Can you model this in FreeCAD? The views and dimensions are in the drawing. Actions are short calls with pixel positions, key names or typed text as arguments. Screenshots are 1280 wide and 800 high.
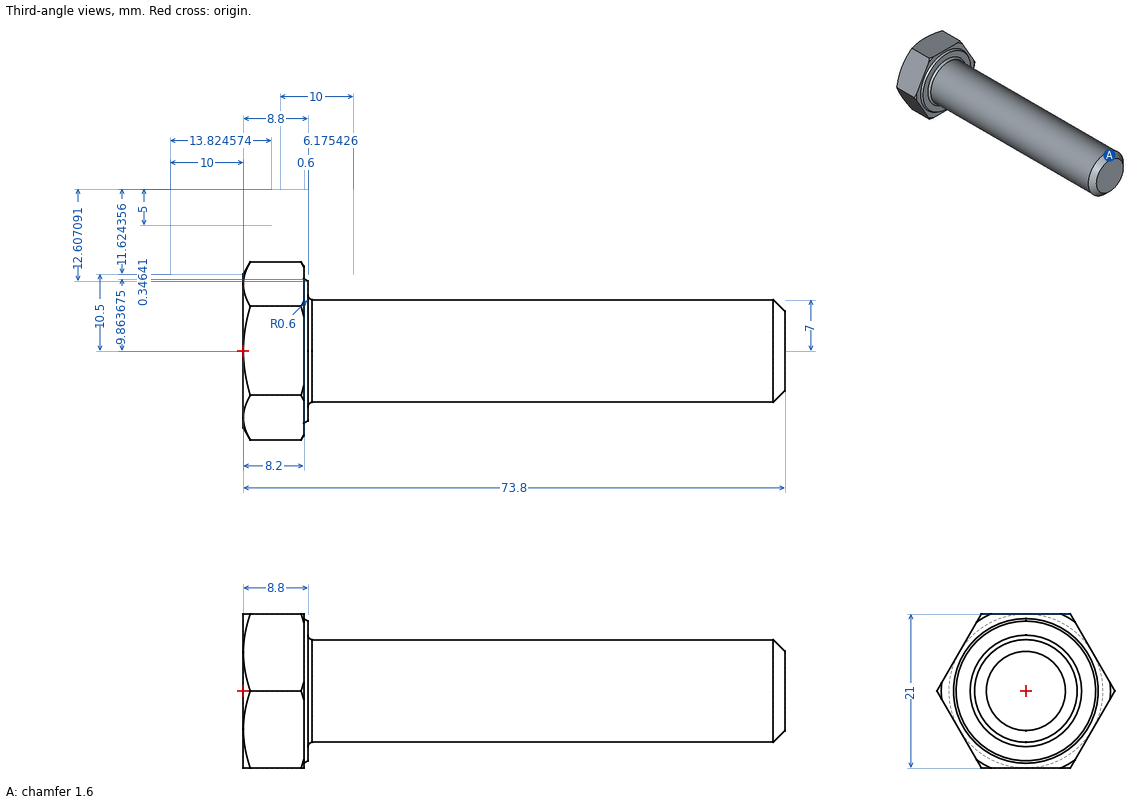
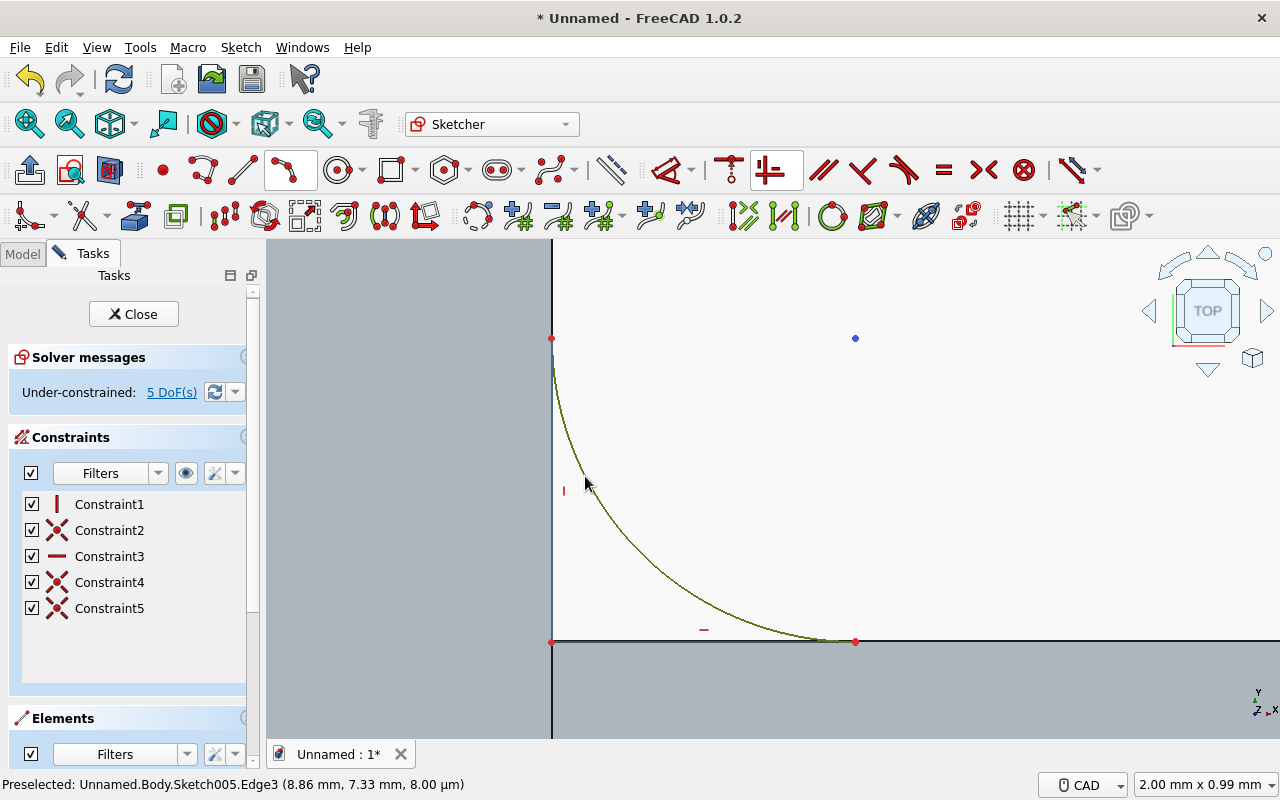
click(904, 170)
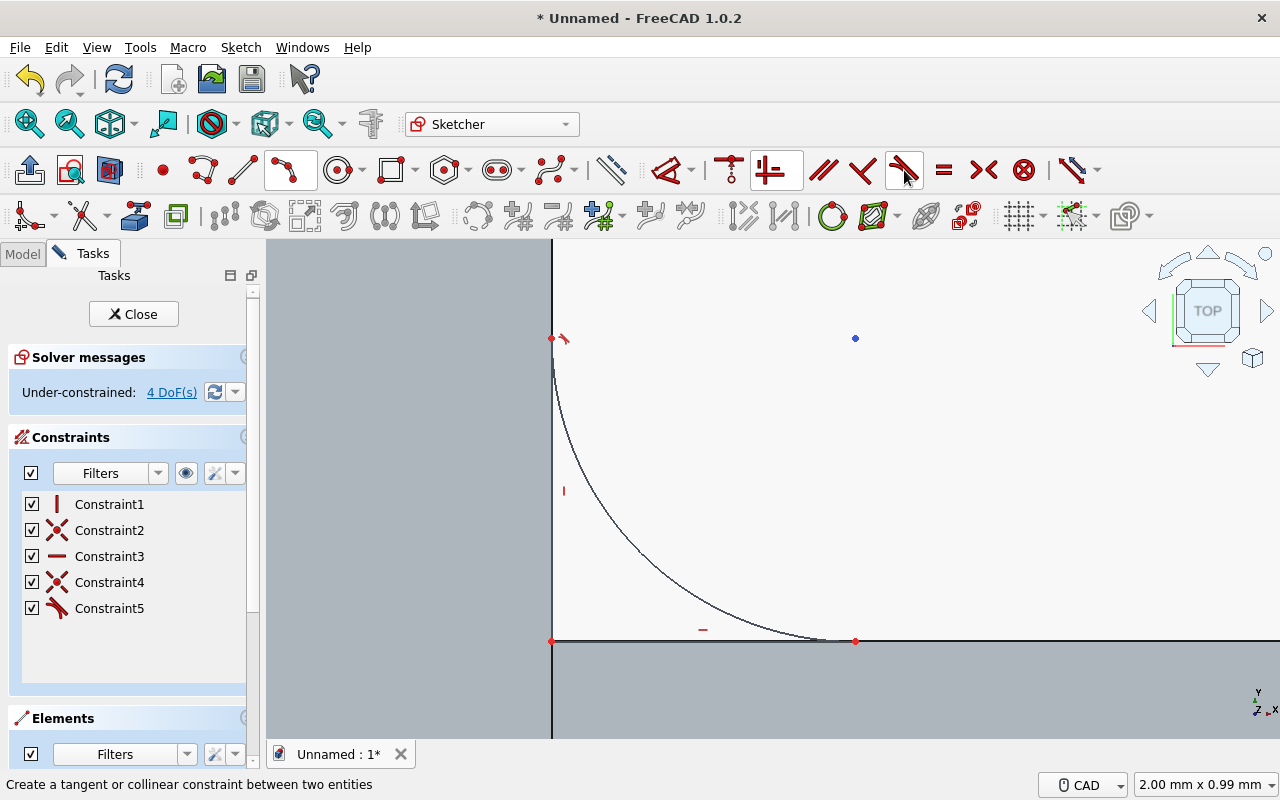
click(643, 642)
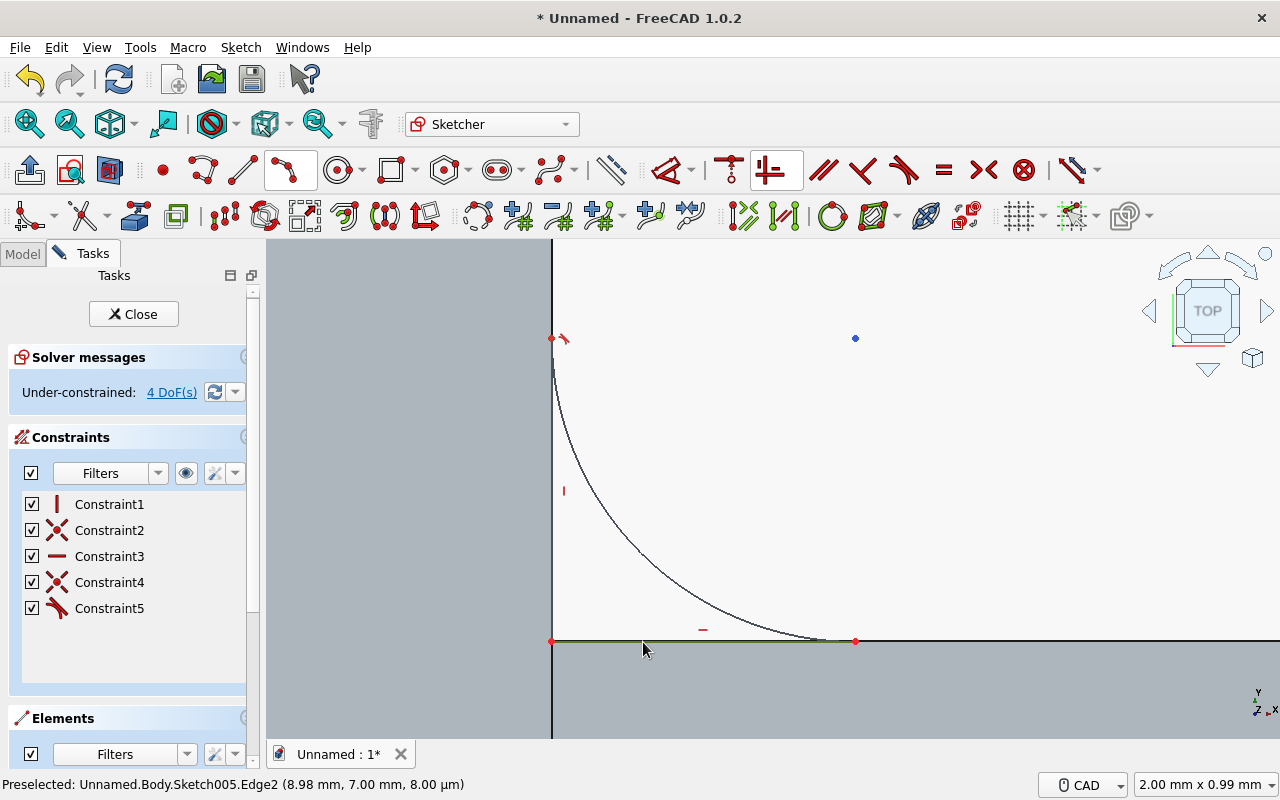
click(585, 476)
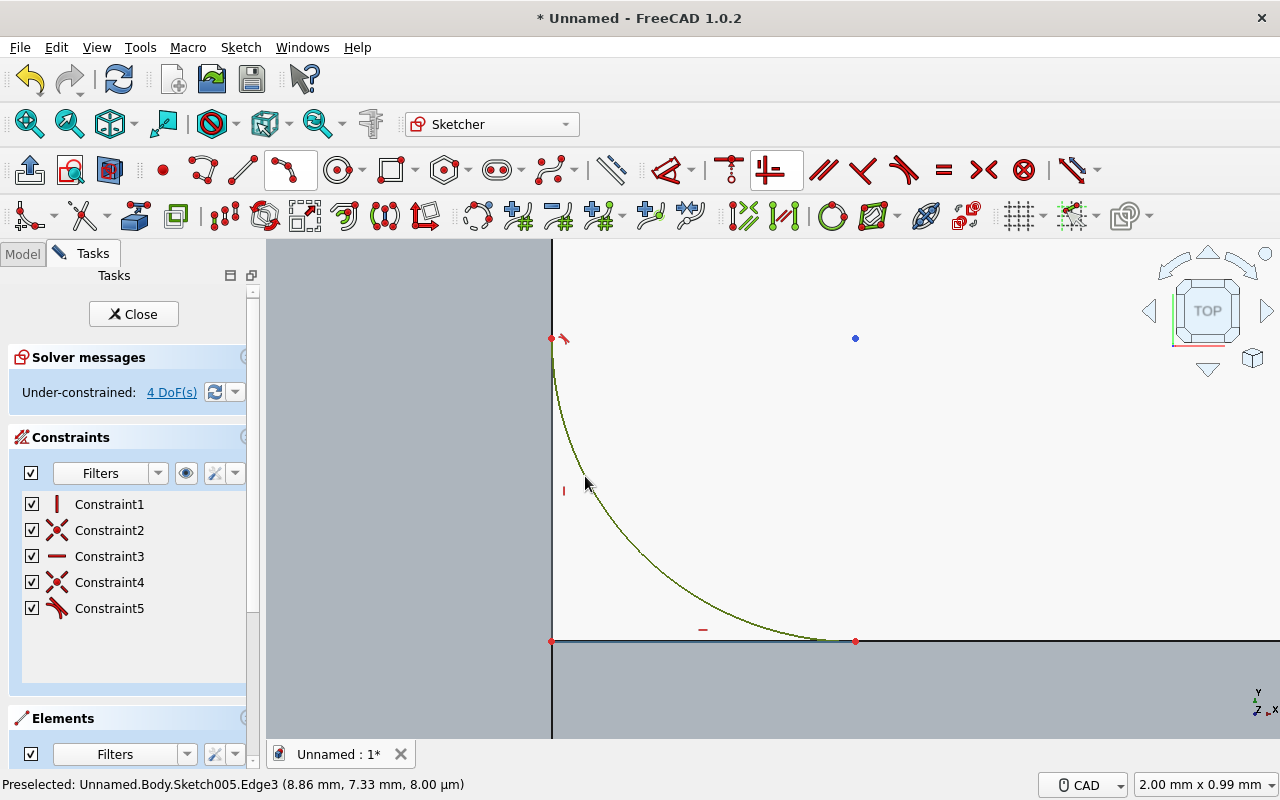
click(904, 170)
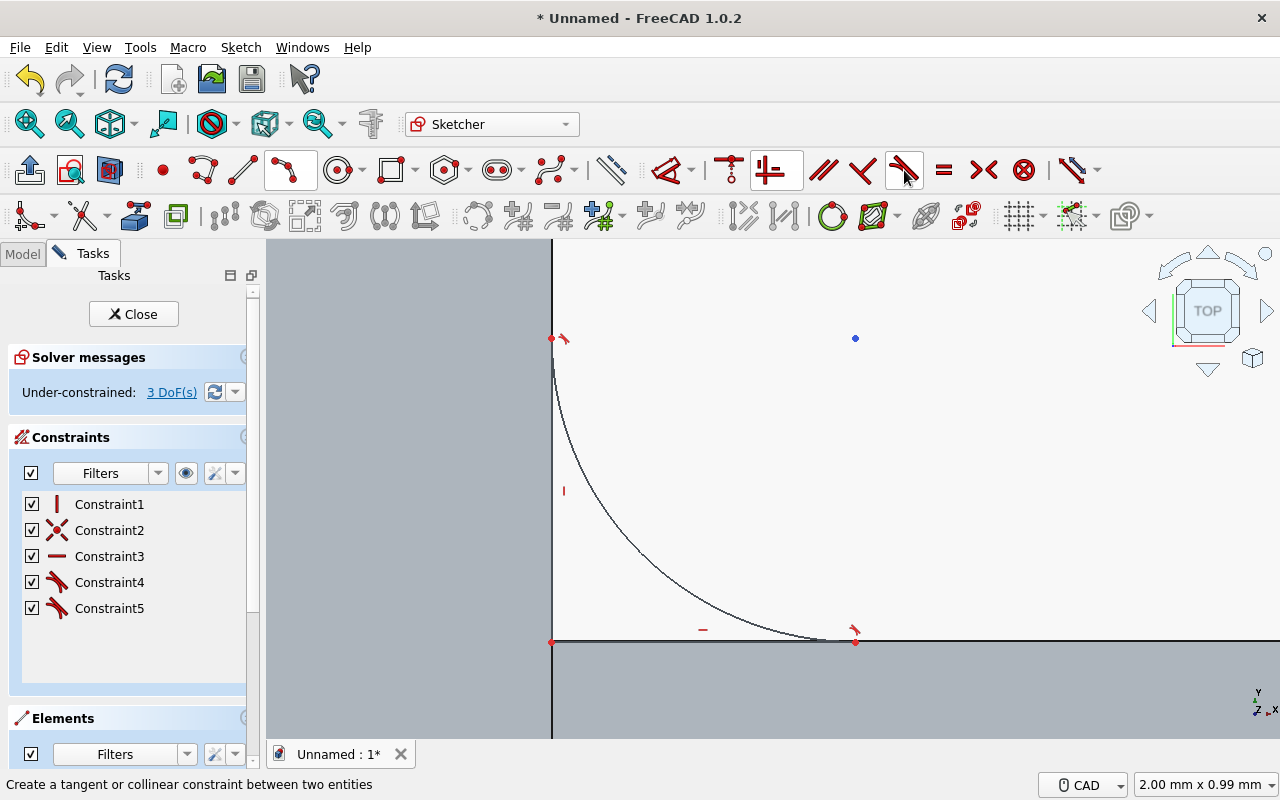
click(666, 170)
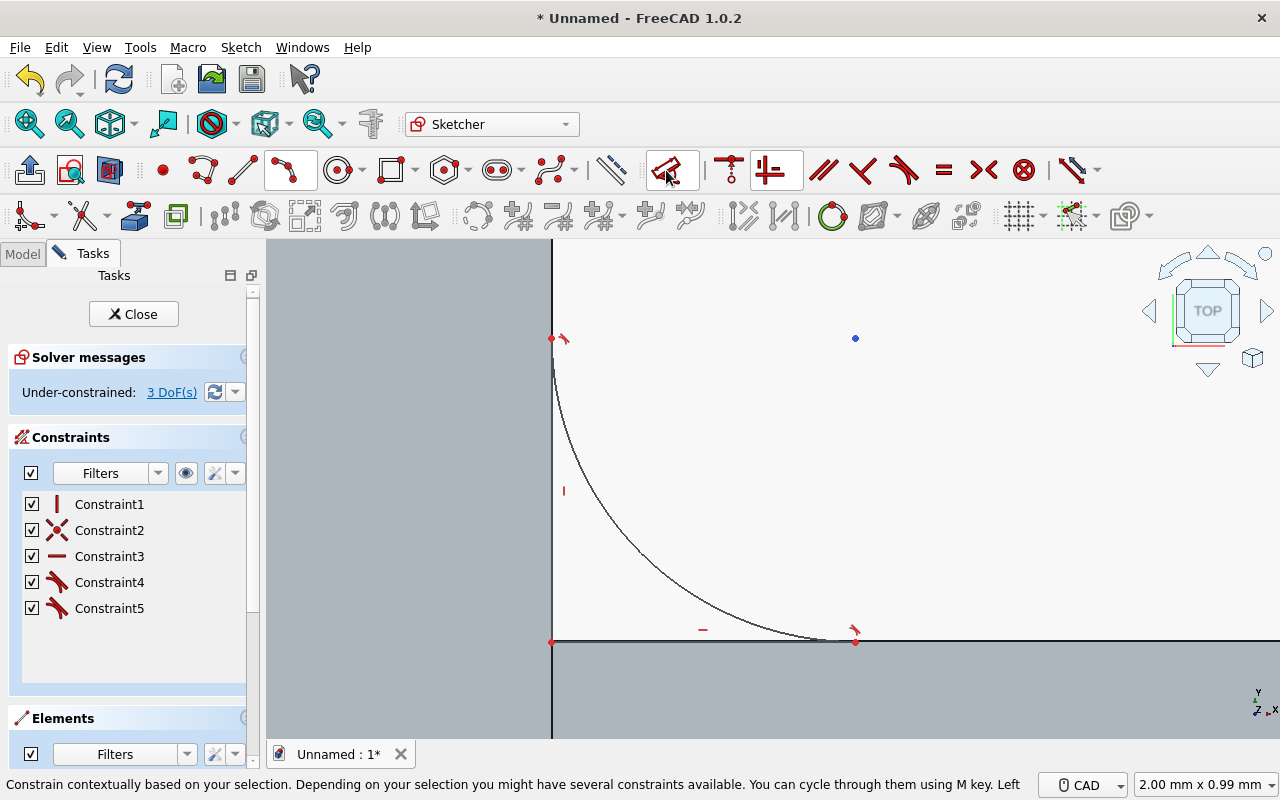
click(585, 476)
click(520, 328)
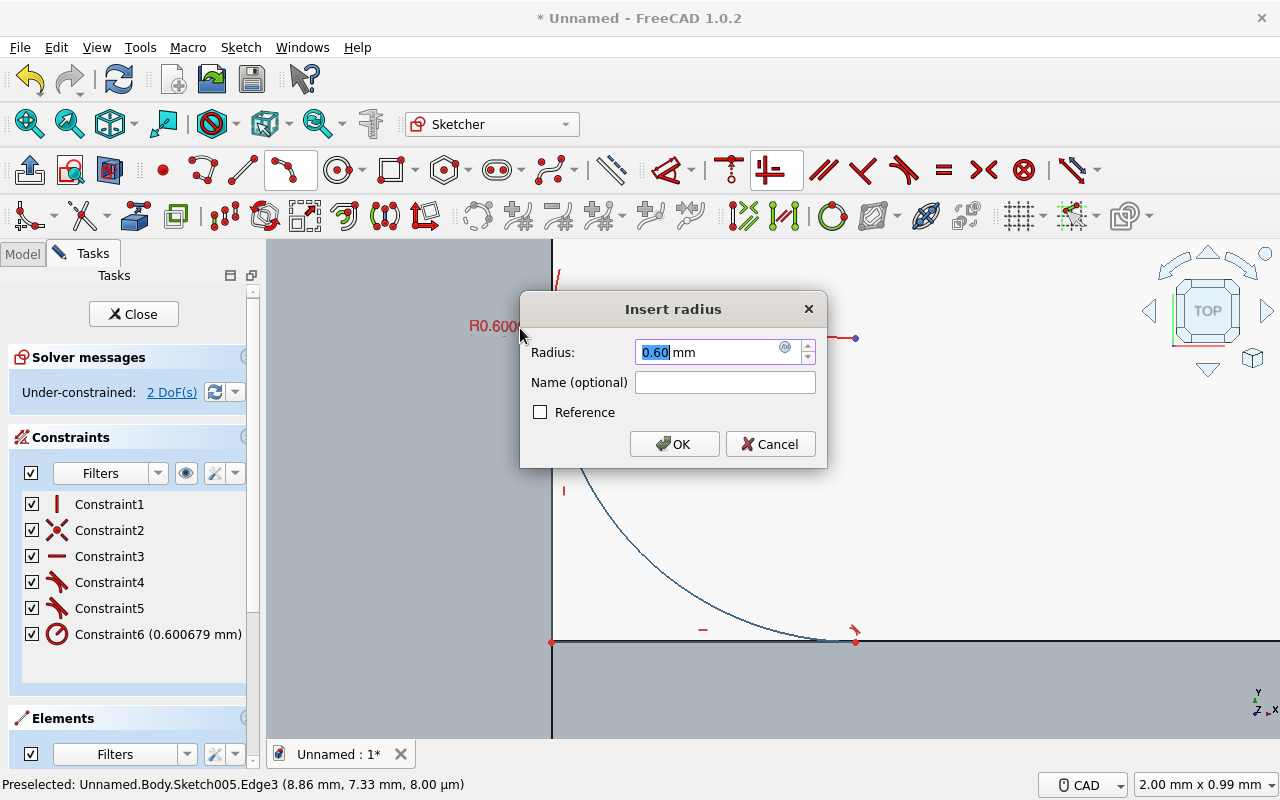
text(0.6)
key(Return)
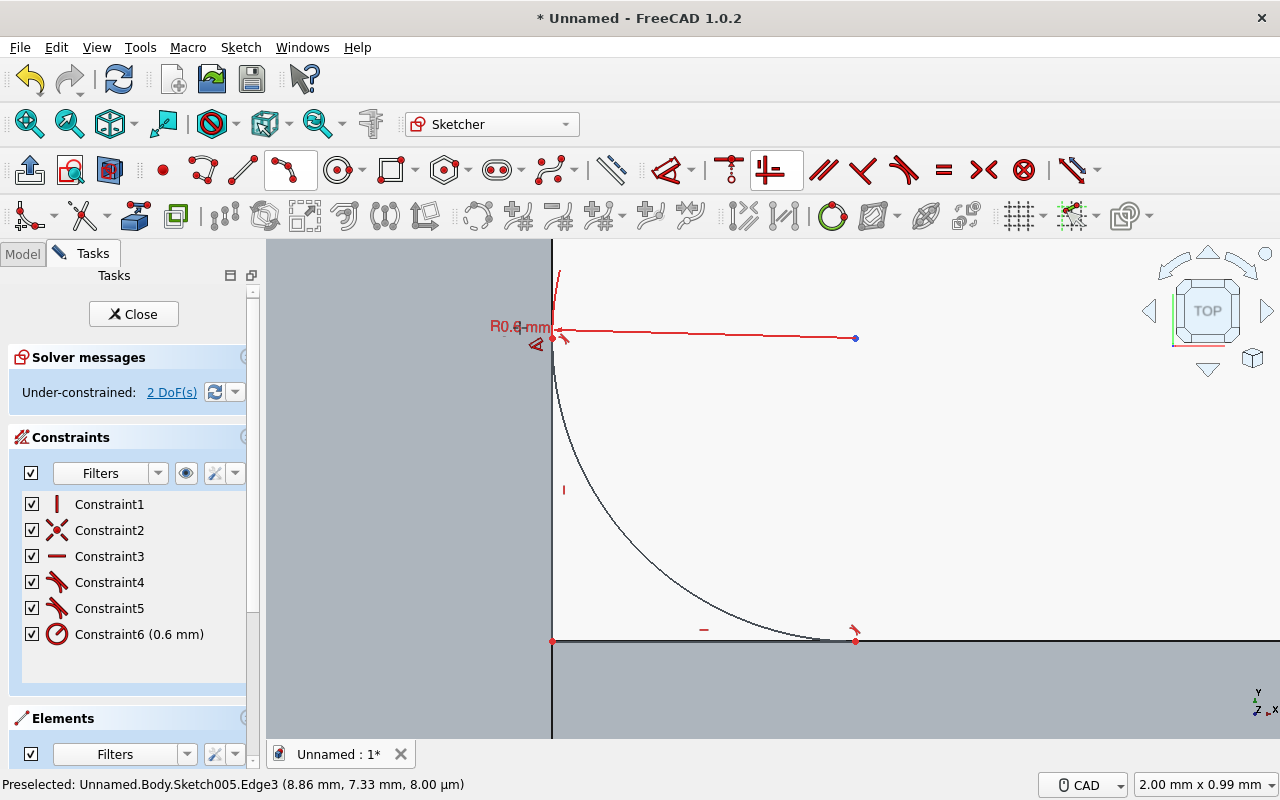
click(552, 642)
click(586, 676)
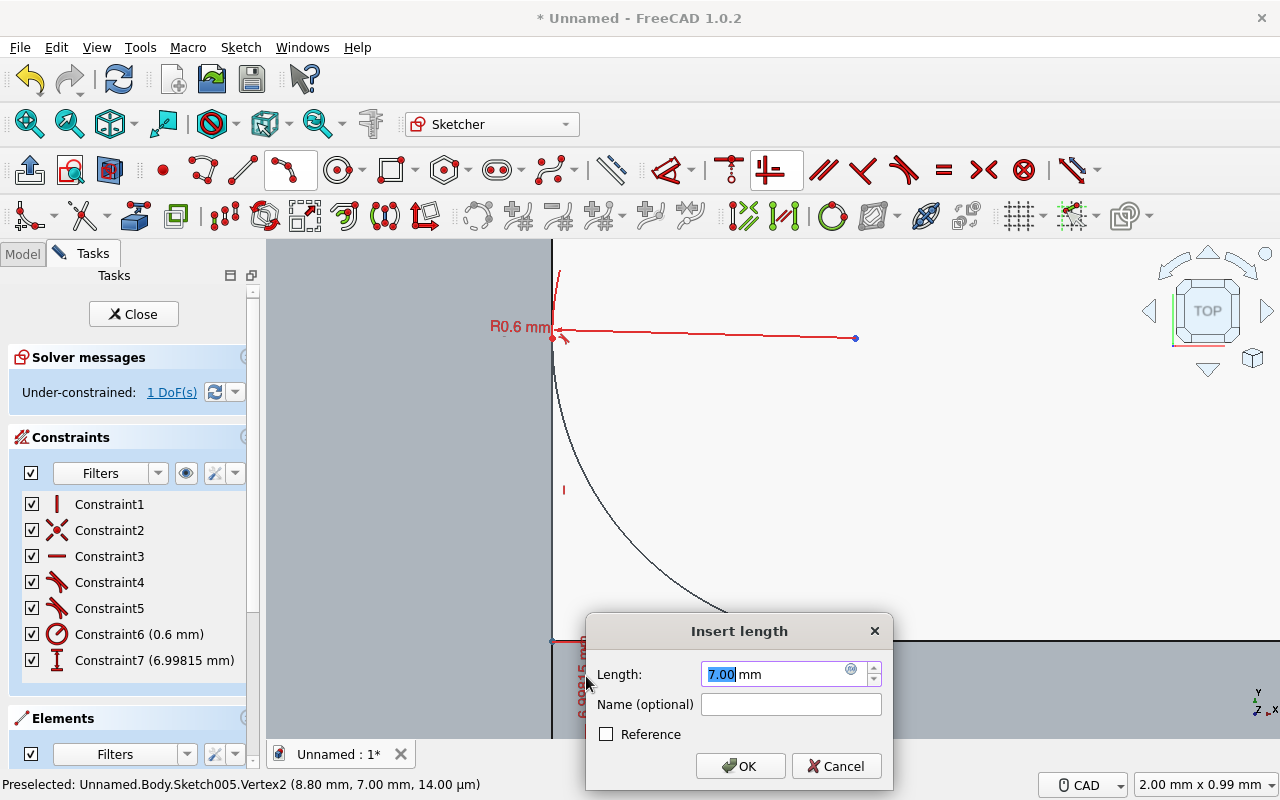
text(7)
key(Return)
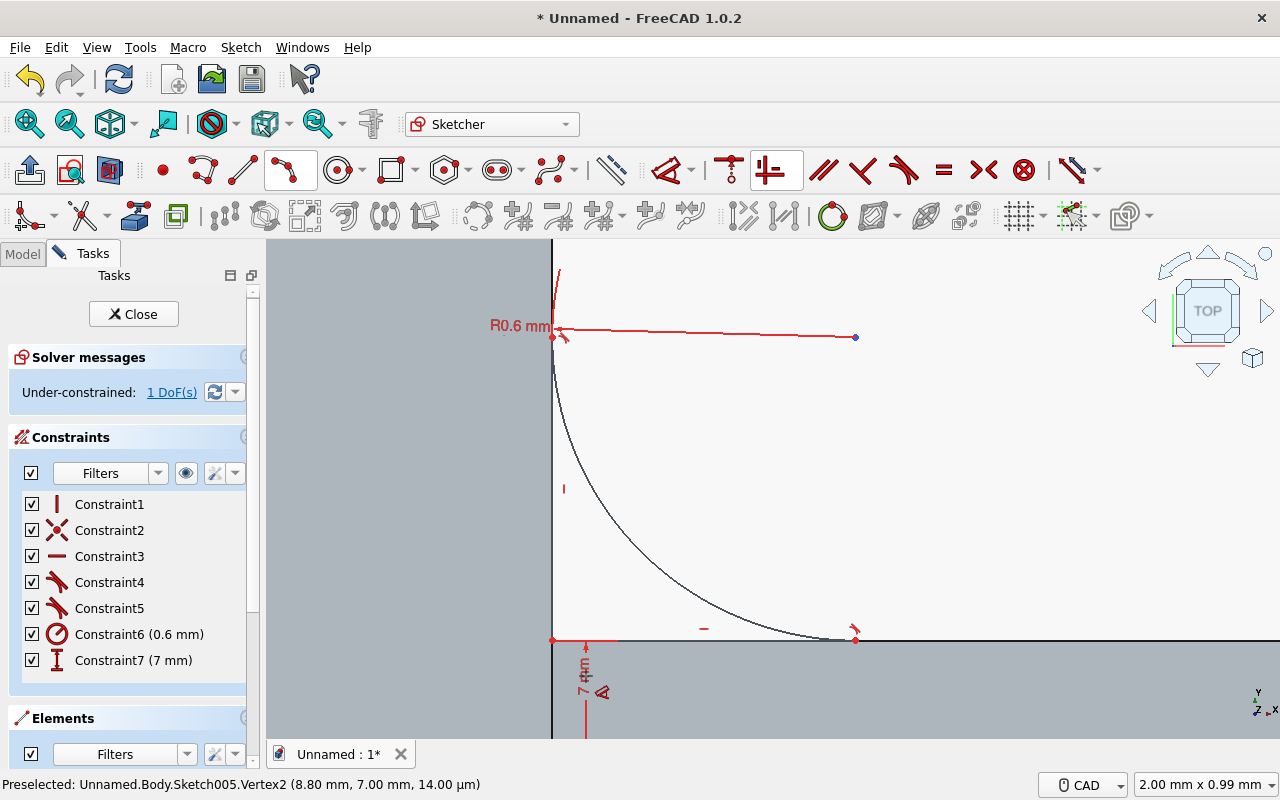
click(552, 337)
click(423, 303)